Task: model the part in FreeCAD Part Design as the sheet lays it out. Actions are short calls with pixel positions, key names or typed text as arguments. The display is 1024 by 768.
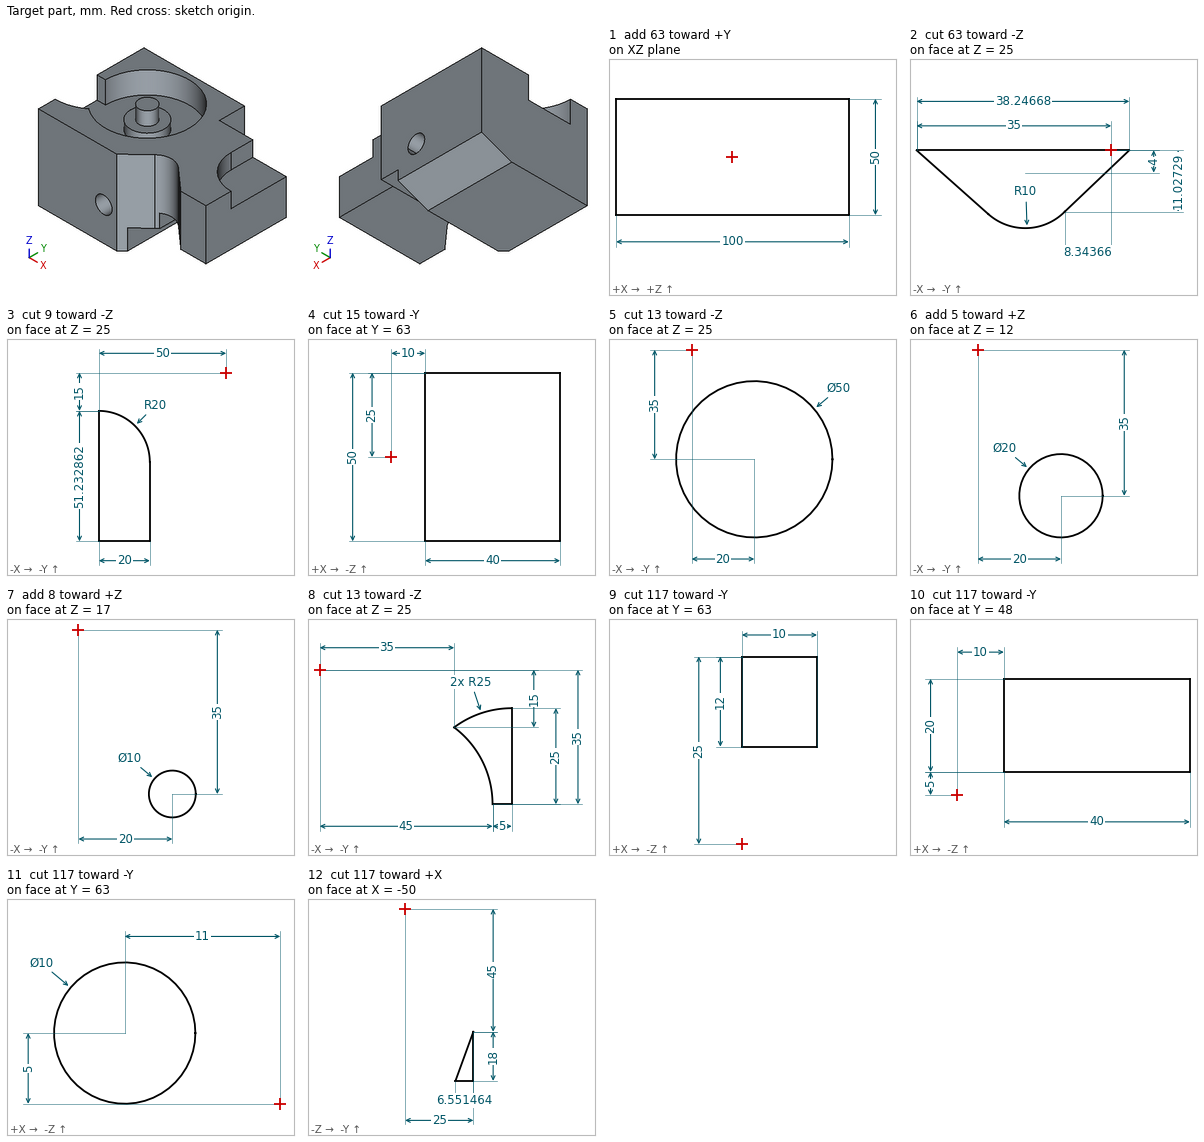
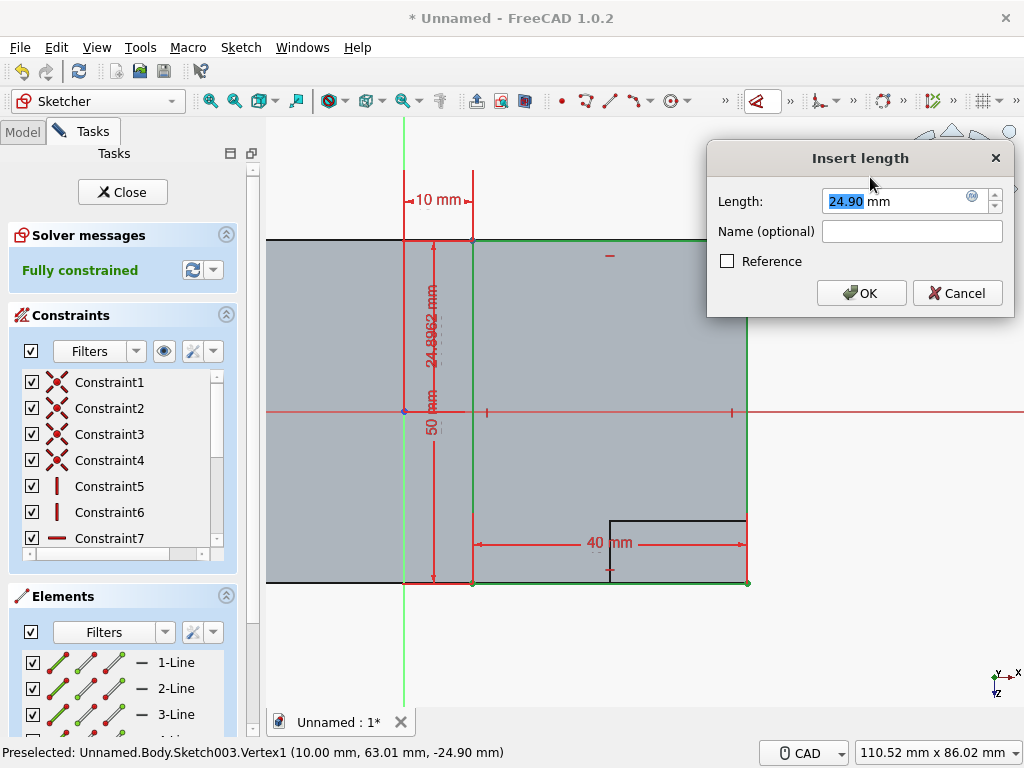
text(25)
key(Return)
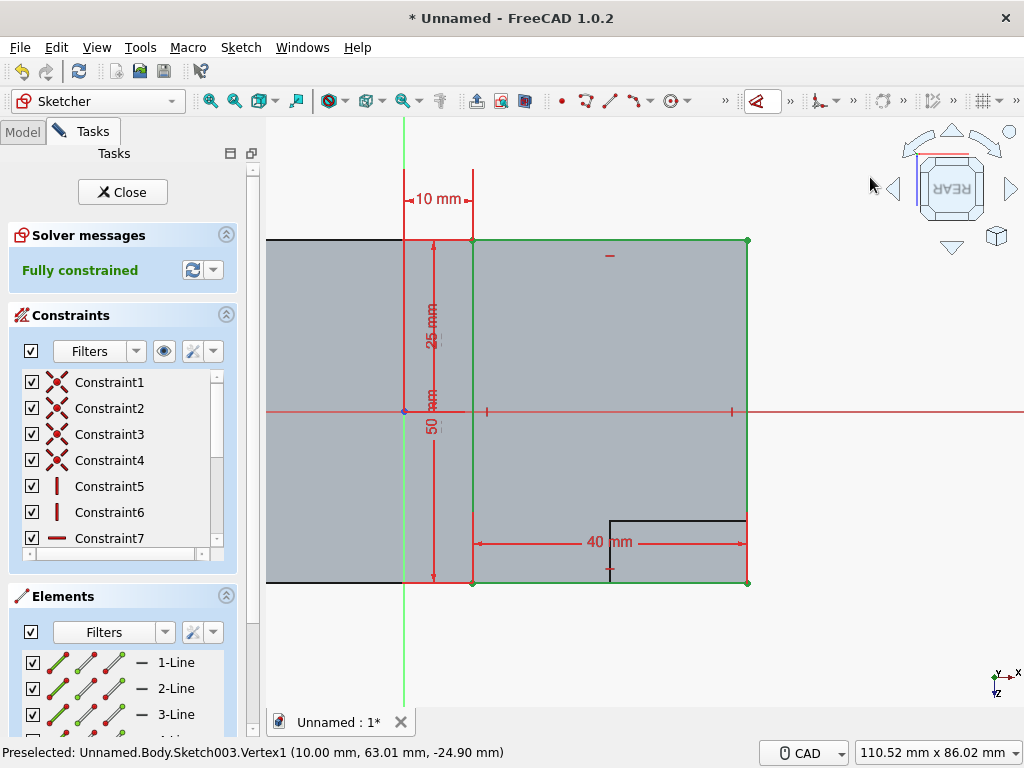
click(123, 192)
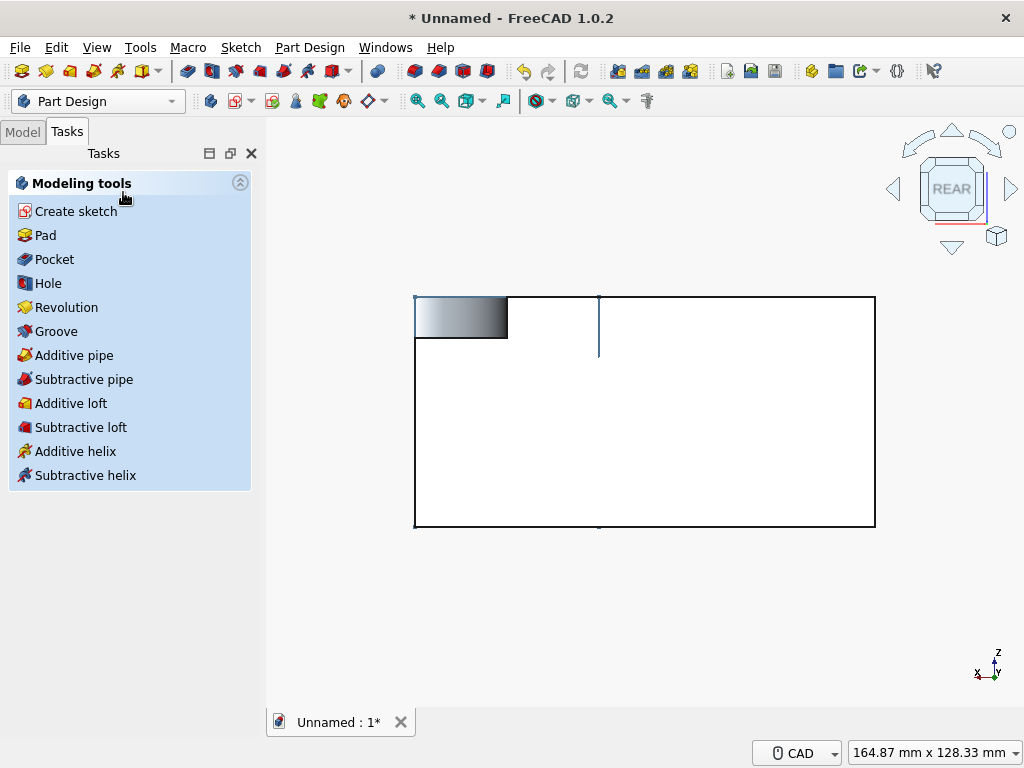
click(188, 72)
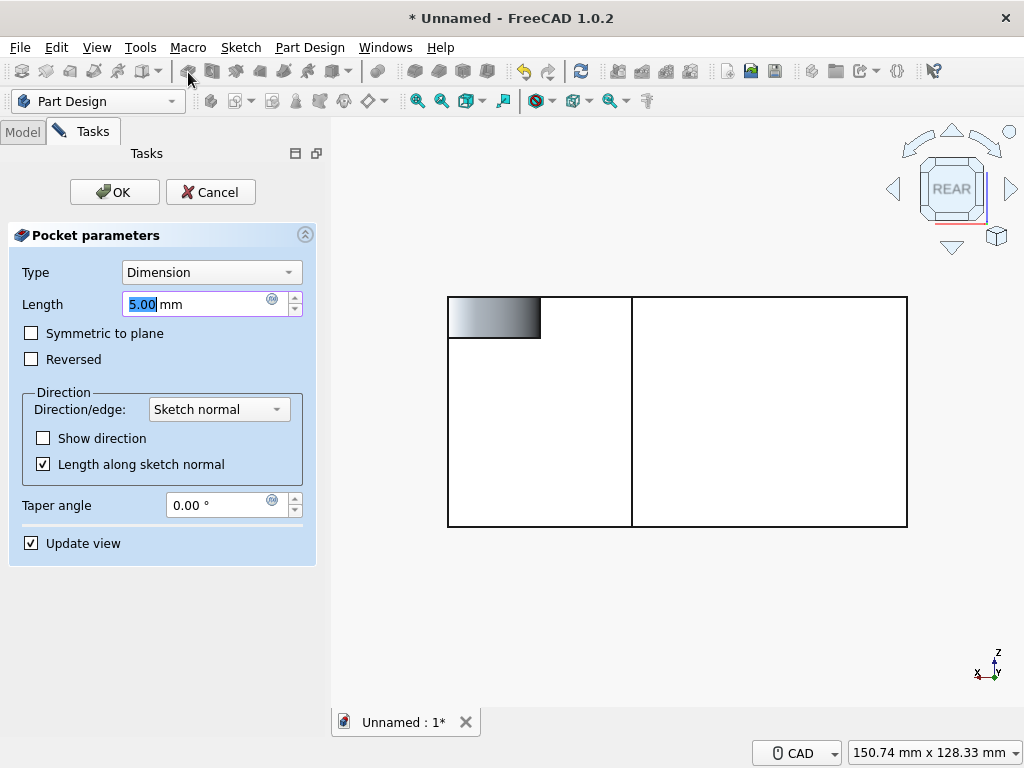
text(15)
key(Tab)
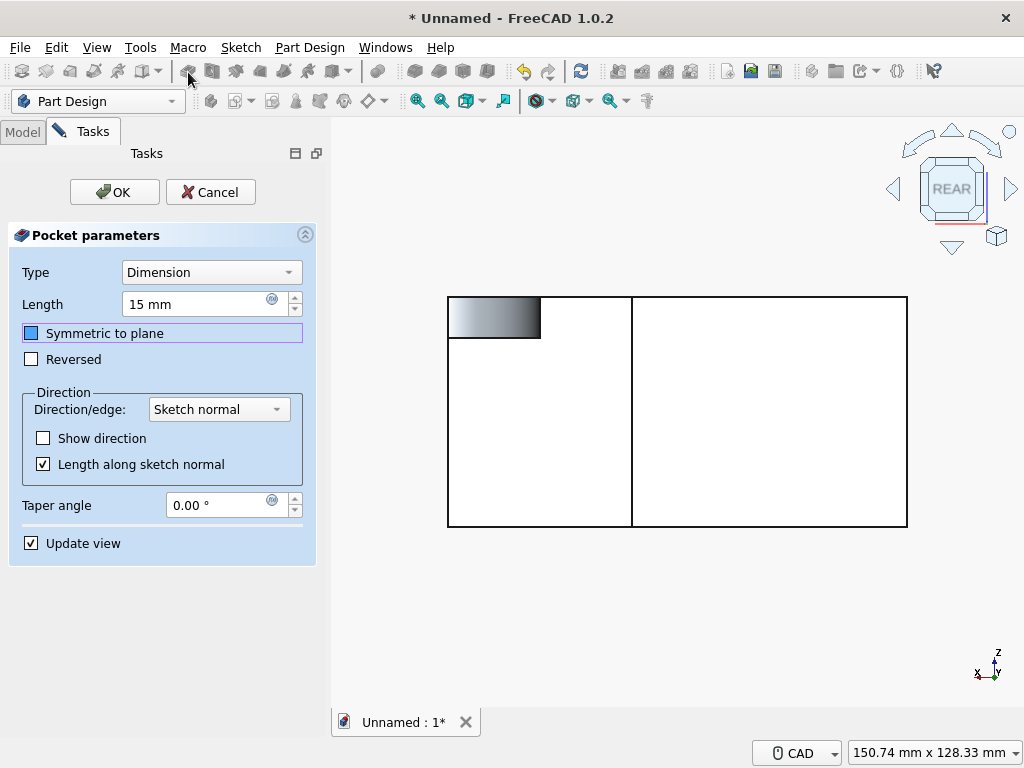
click(115, 192)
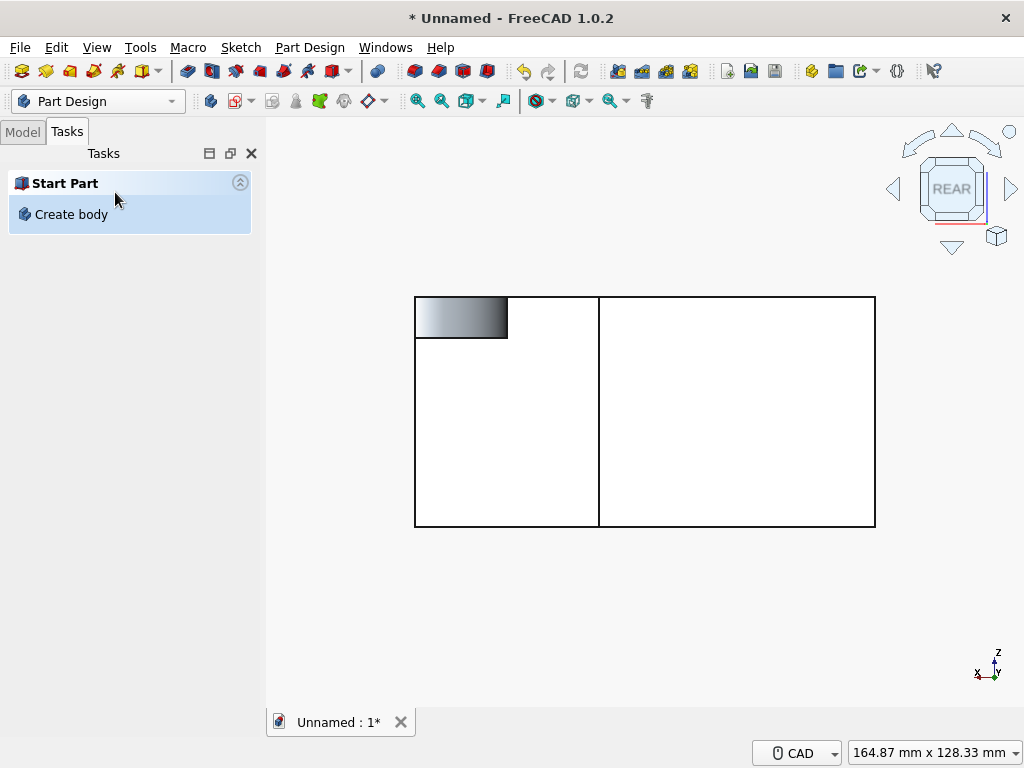
key(0)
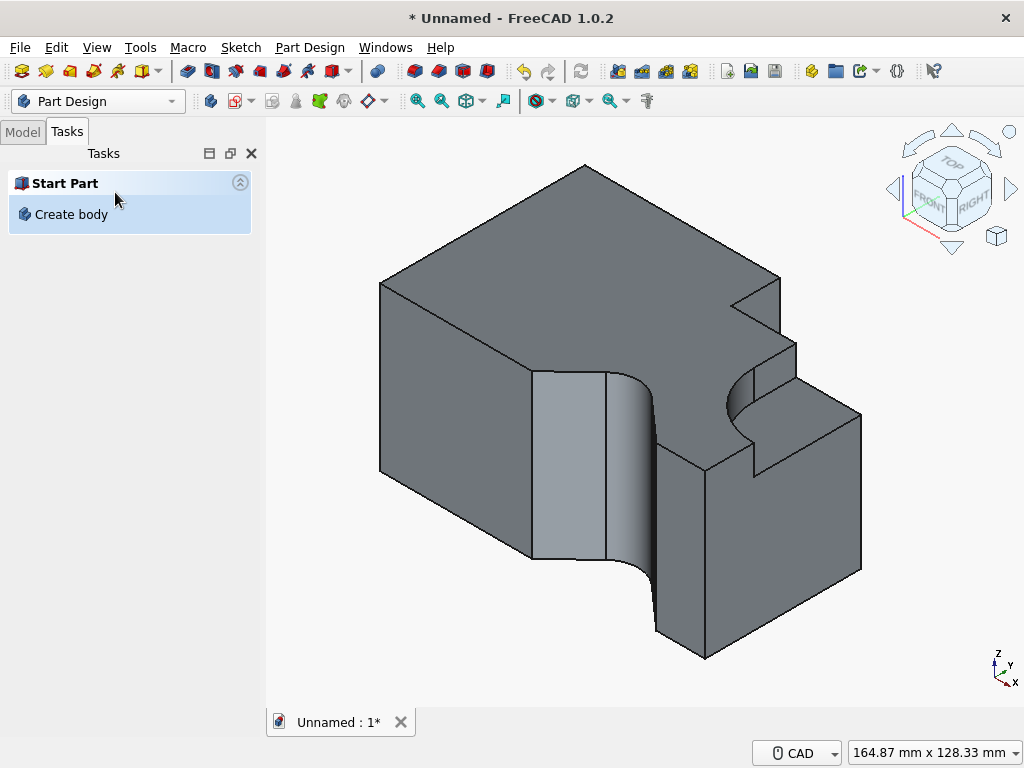
click(599, 290)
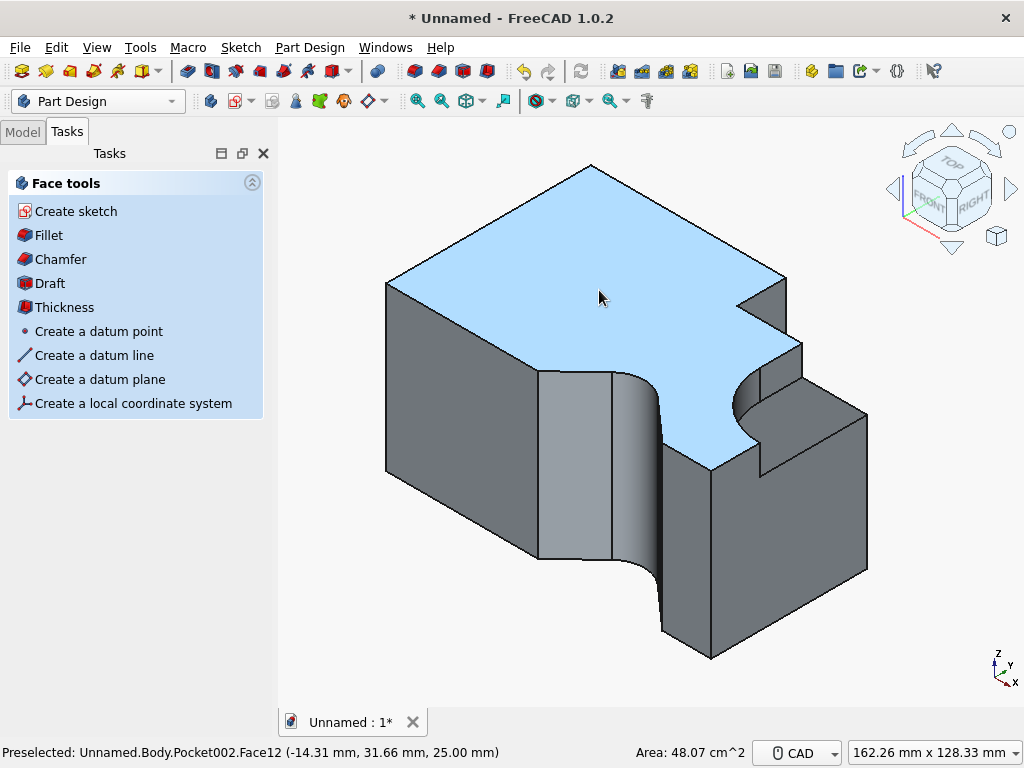
click(236, 102)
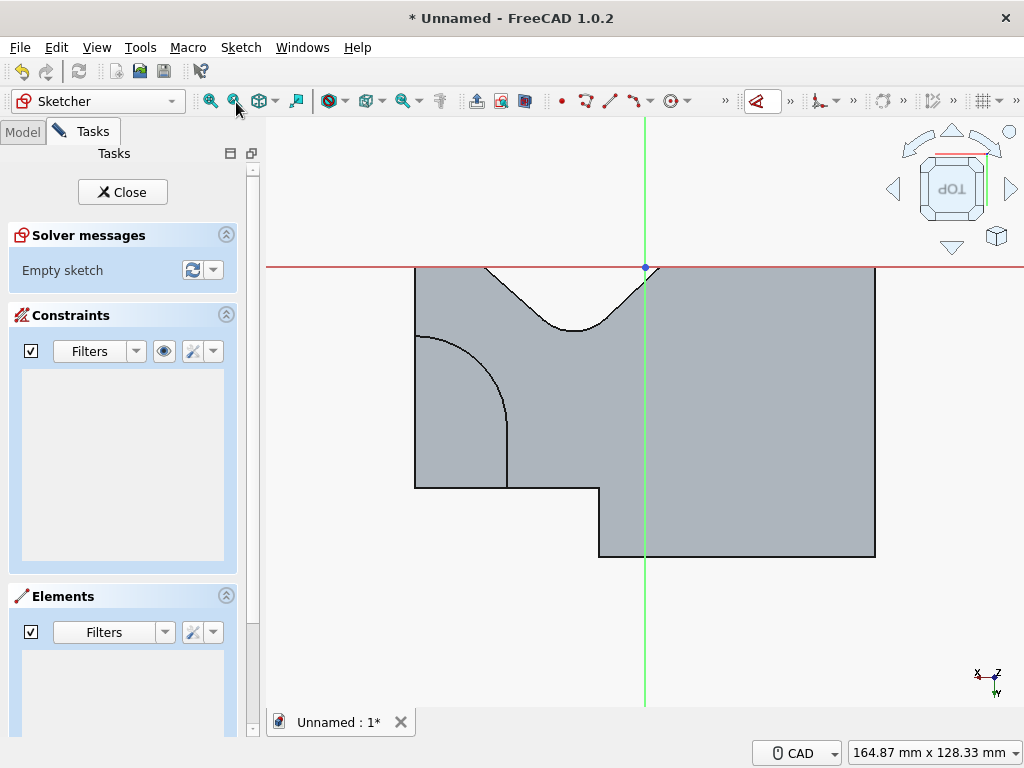
scroll(294, 443, down, 1)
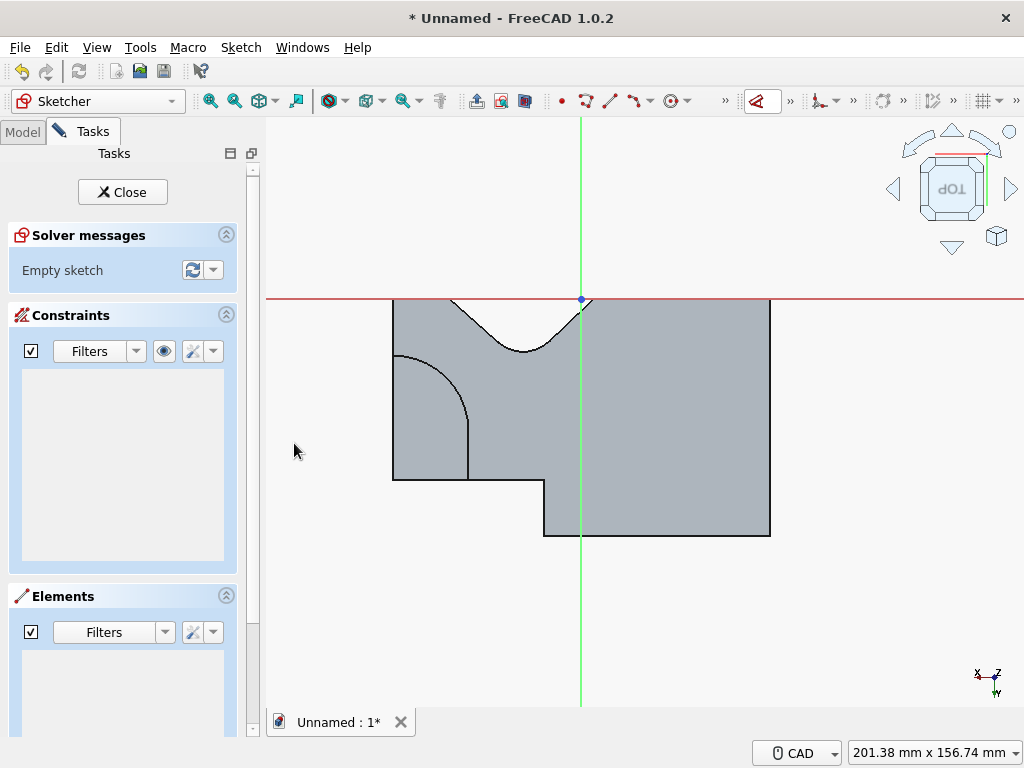
scroll(754, 412, up, 3)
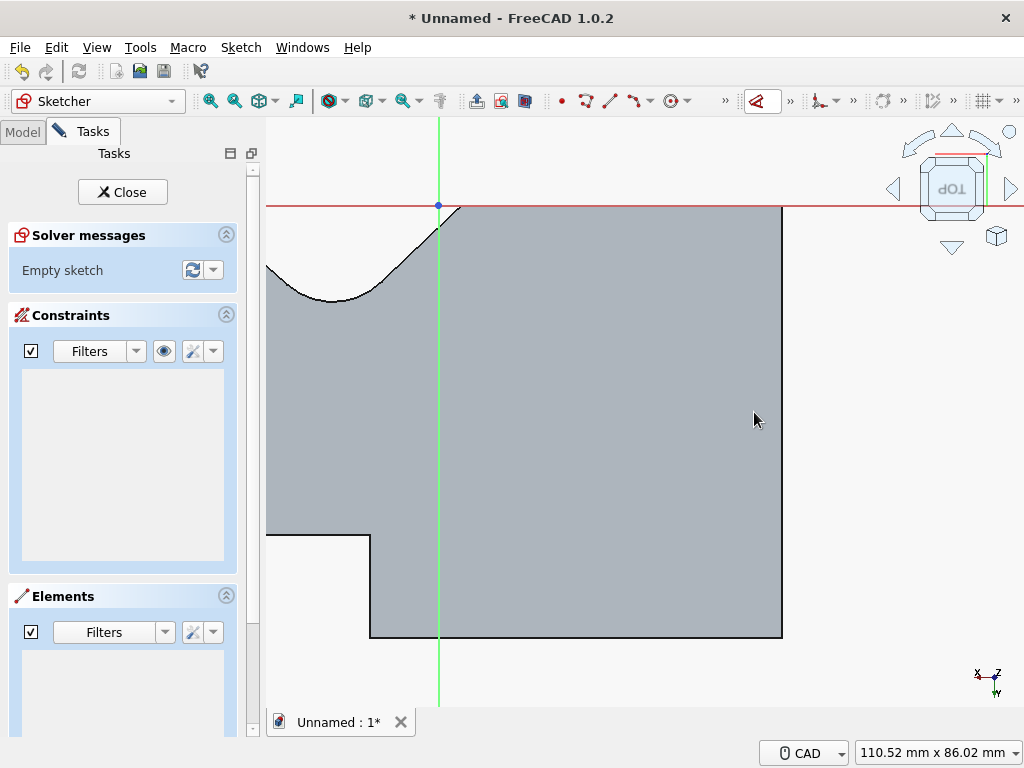
click(672, 102)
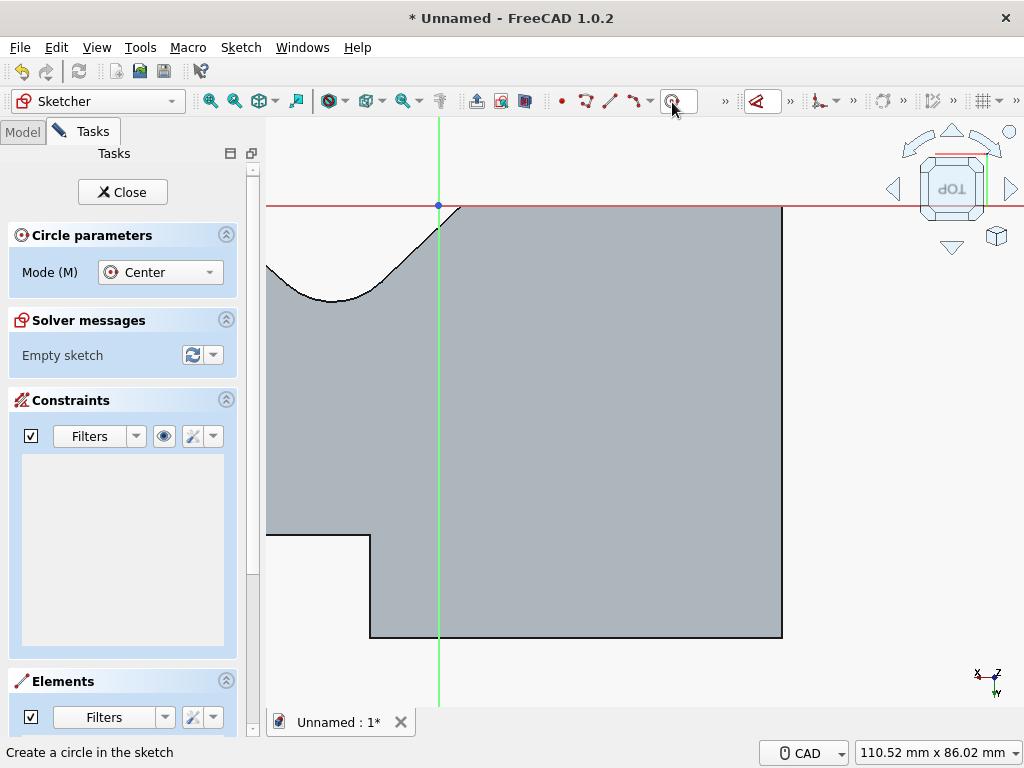
click(576, 446)
click(697, 325)
key(Escape)